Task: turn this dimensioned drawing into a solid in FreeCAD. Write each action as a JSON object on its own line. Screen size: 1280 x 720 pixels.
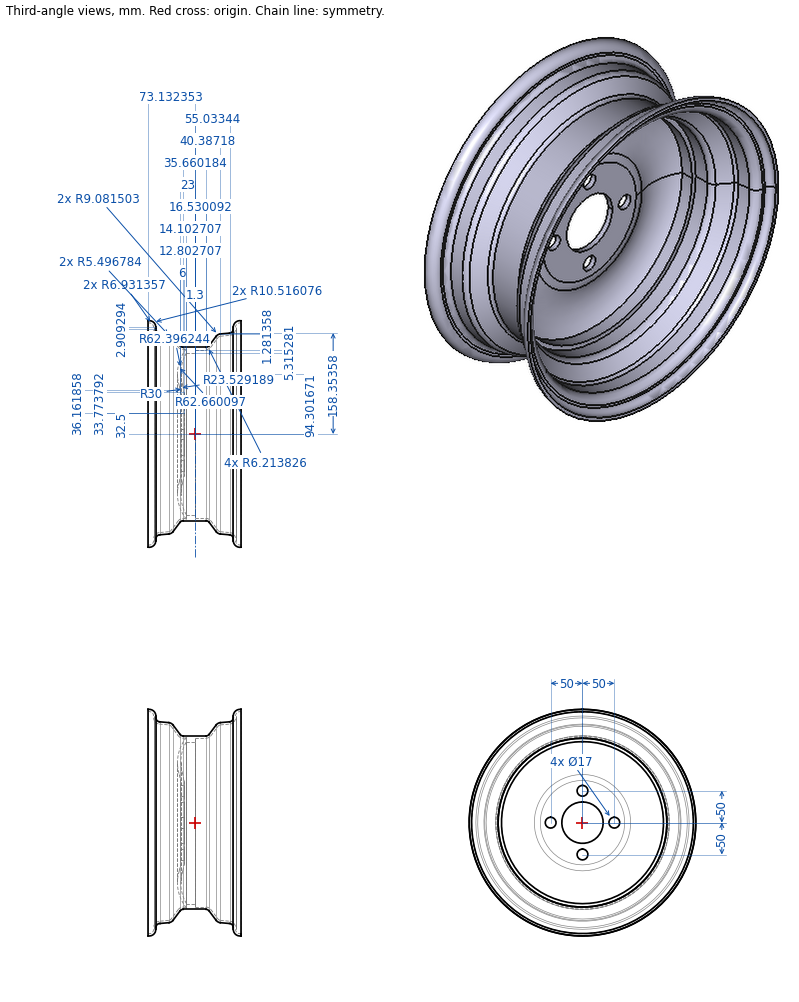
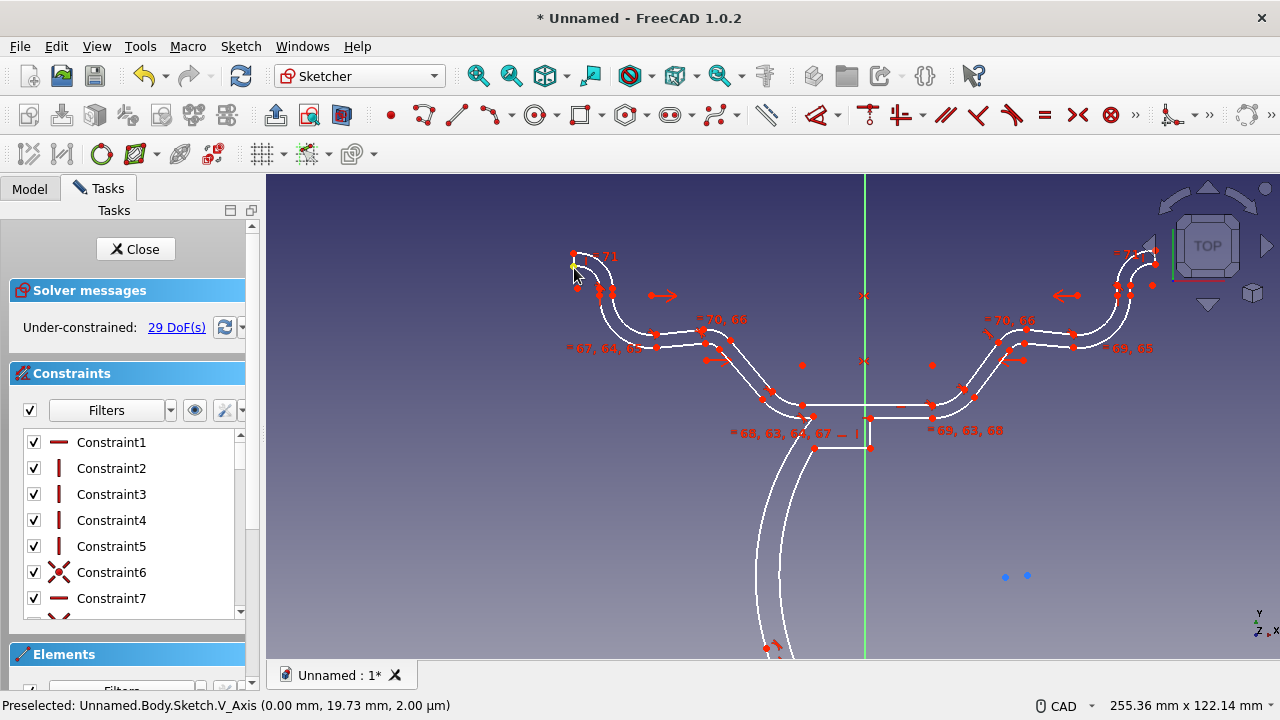
{"action": "left_click", "coordinate": [574, 267]}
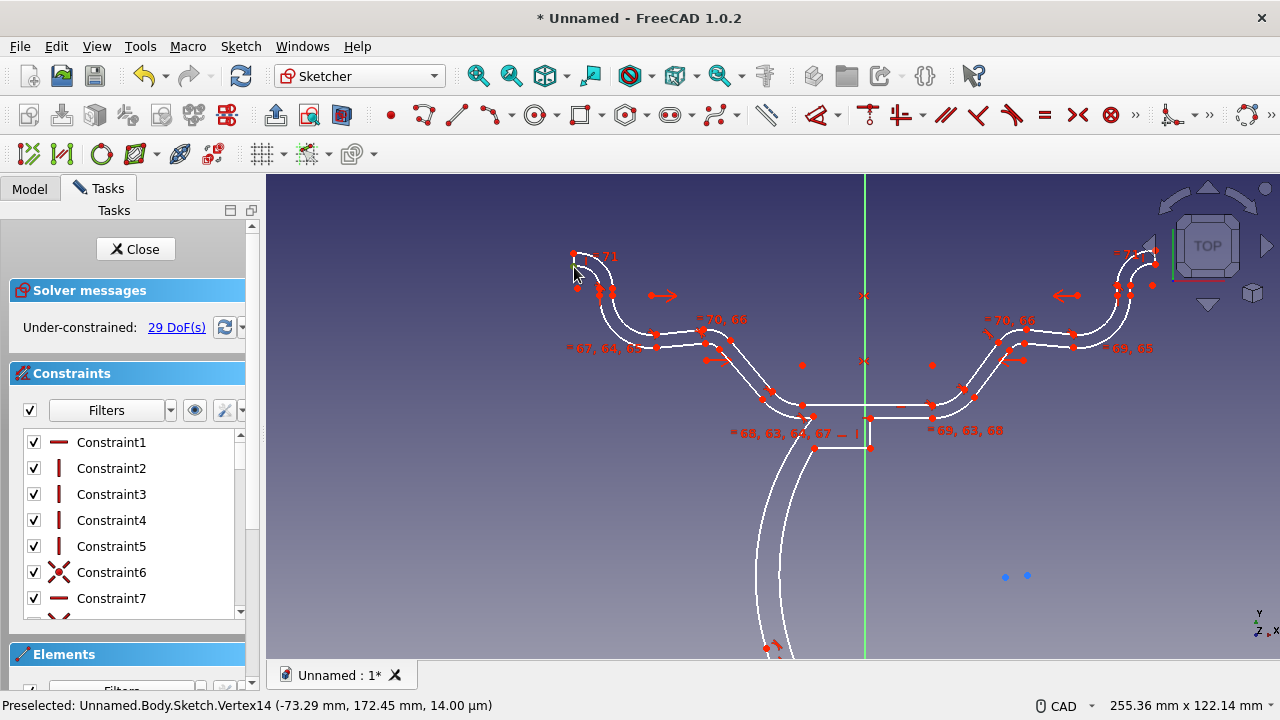
{"action": "scroll", "coordinate": [574, 268], "scroll_direction": "down", "scroll_amount": 4}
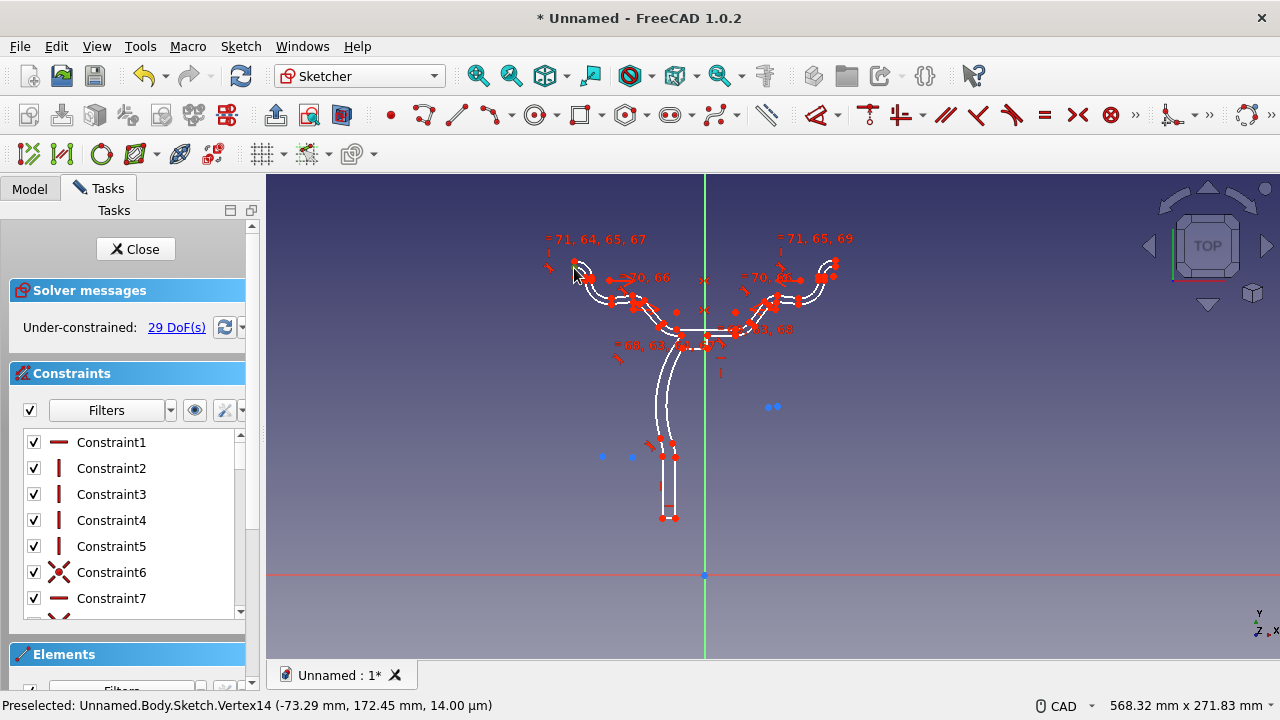
{"action": "scroll", "coordinate": [835, 266], "scroll_direction": "up", "scroll_amount": 4}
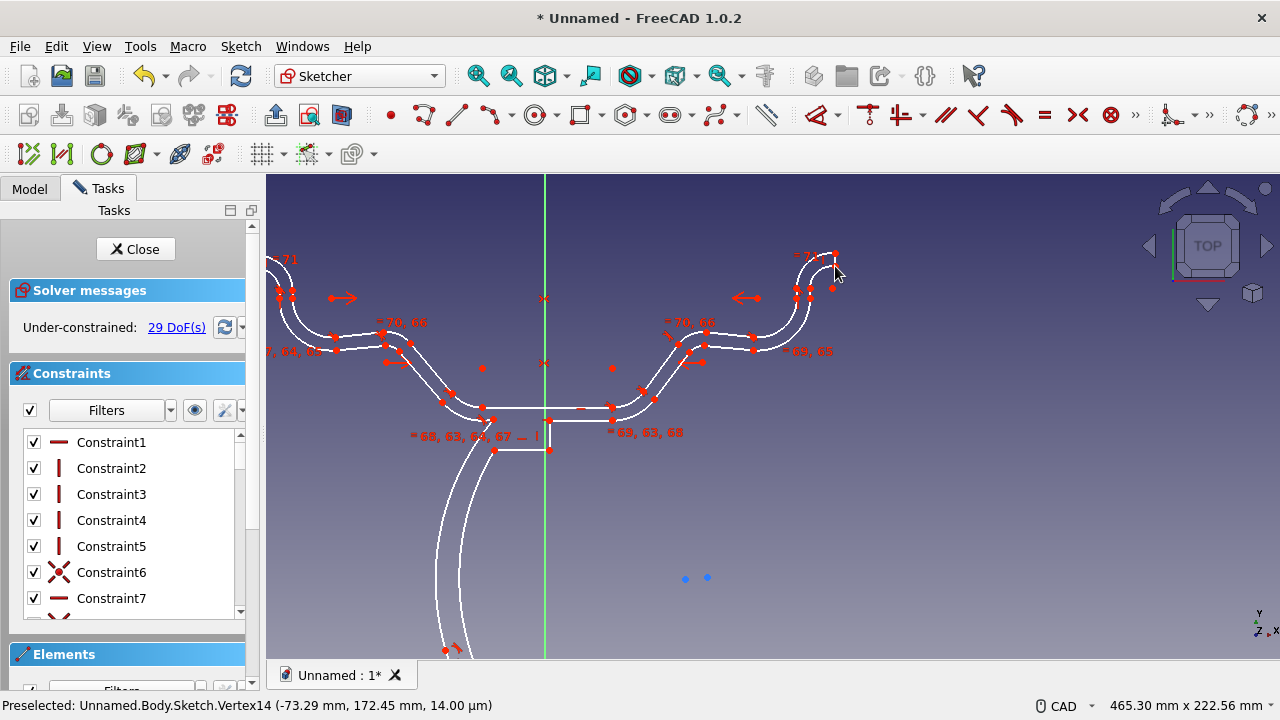
{"action": "left_click", "coordinate": [835, 267]}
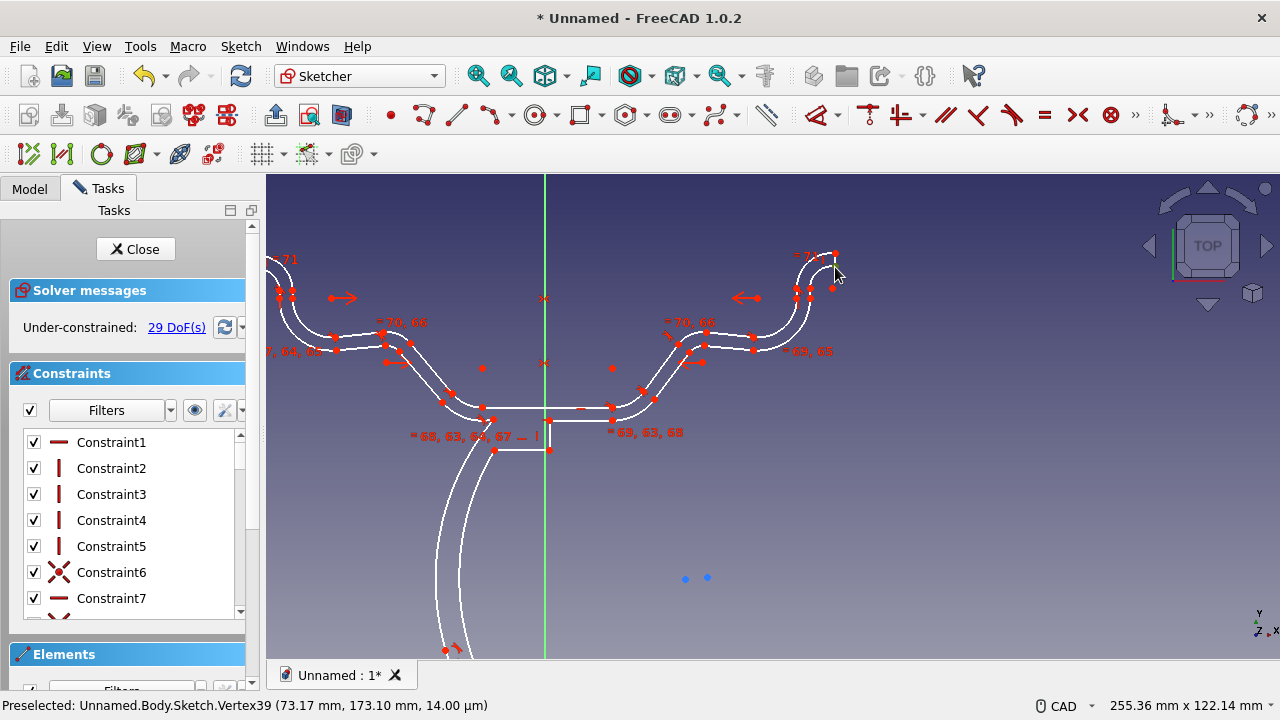
{"action": "left_click", "coordinate": [545, 600]}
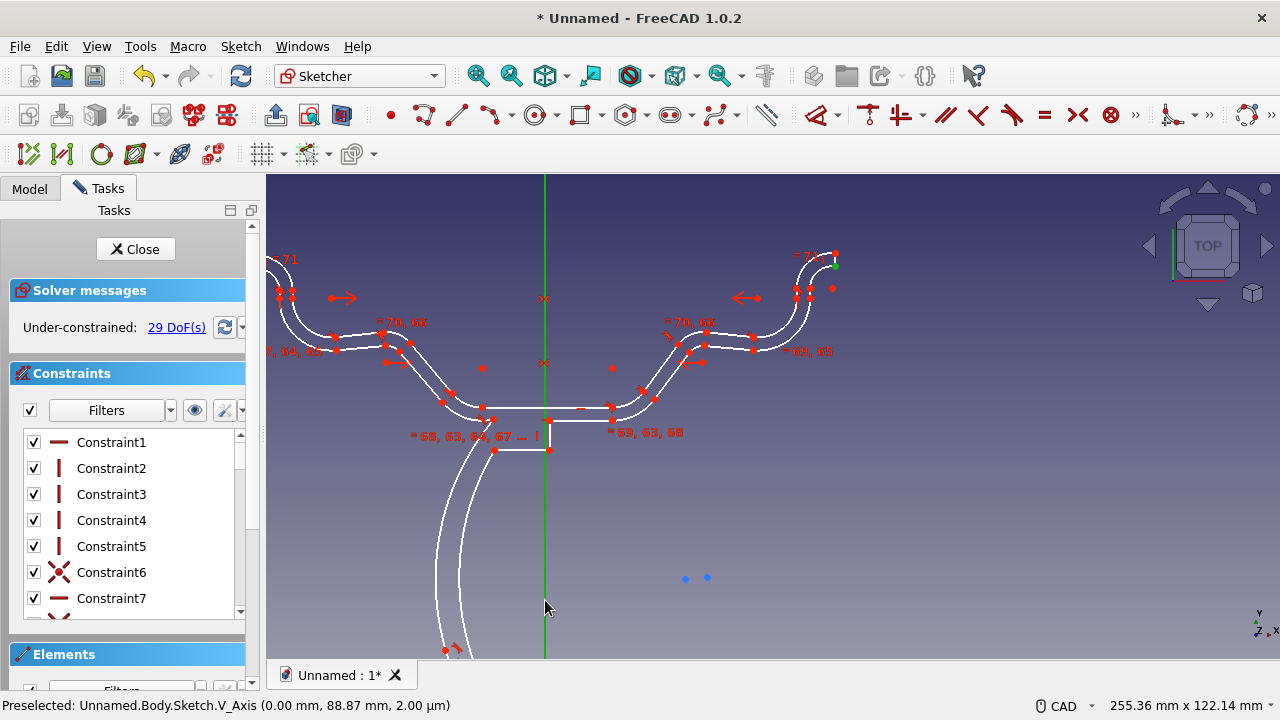
{"action": "key", "text": "s"}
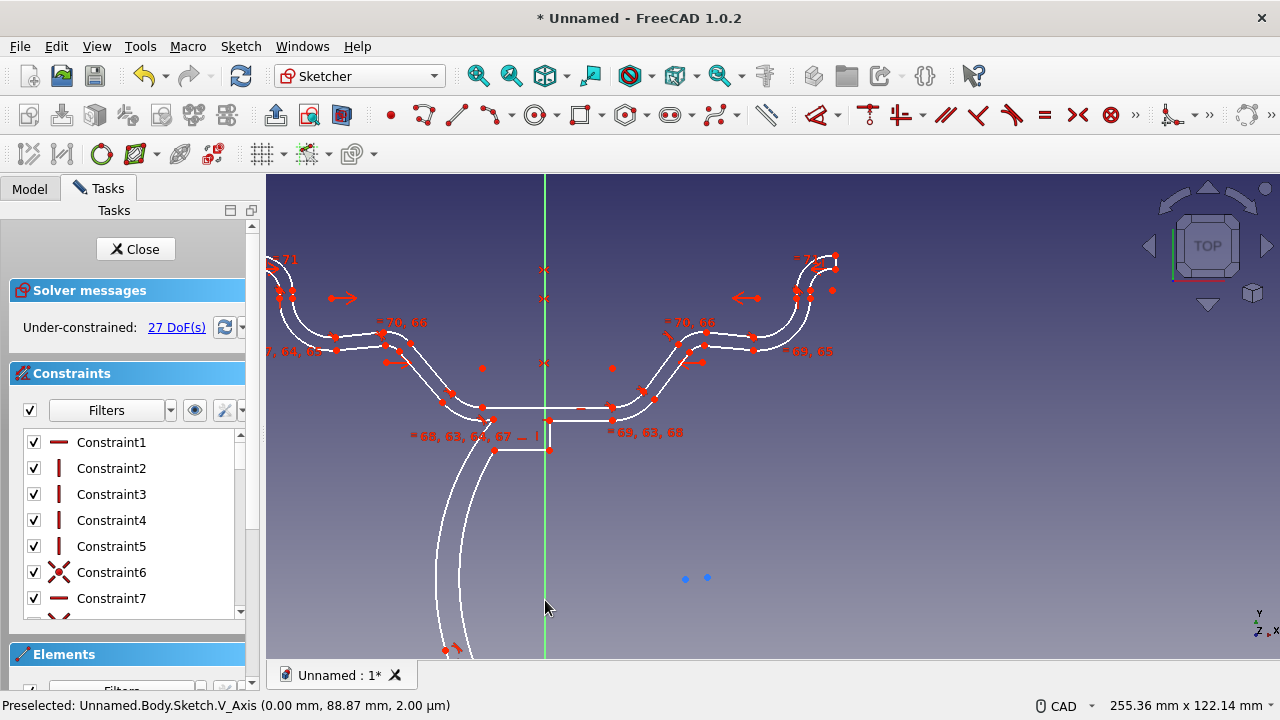
{"action": "left_click", "coordinate": [816, 116]}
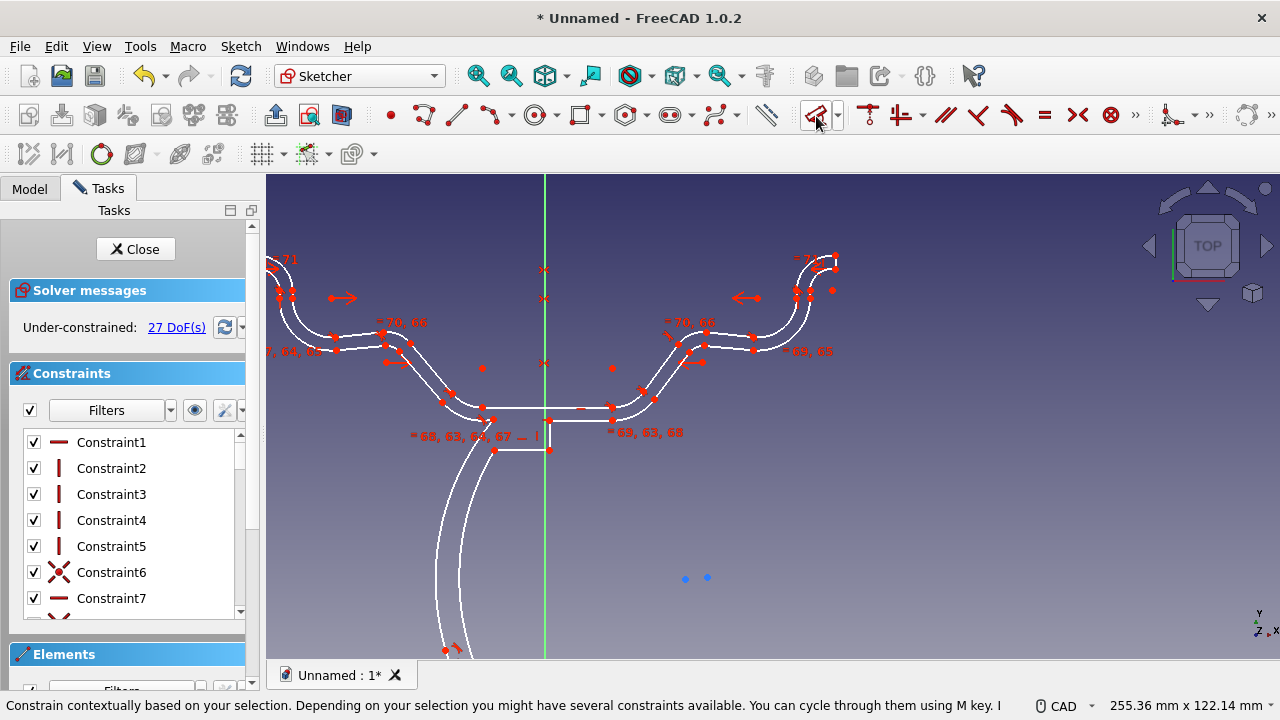
{"action": "scroll", "coordinate": [697, 333], "scroll_direction": "up", "scroll_amount": 2}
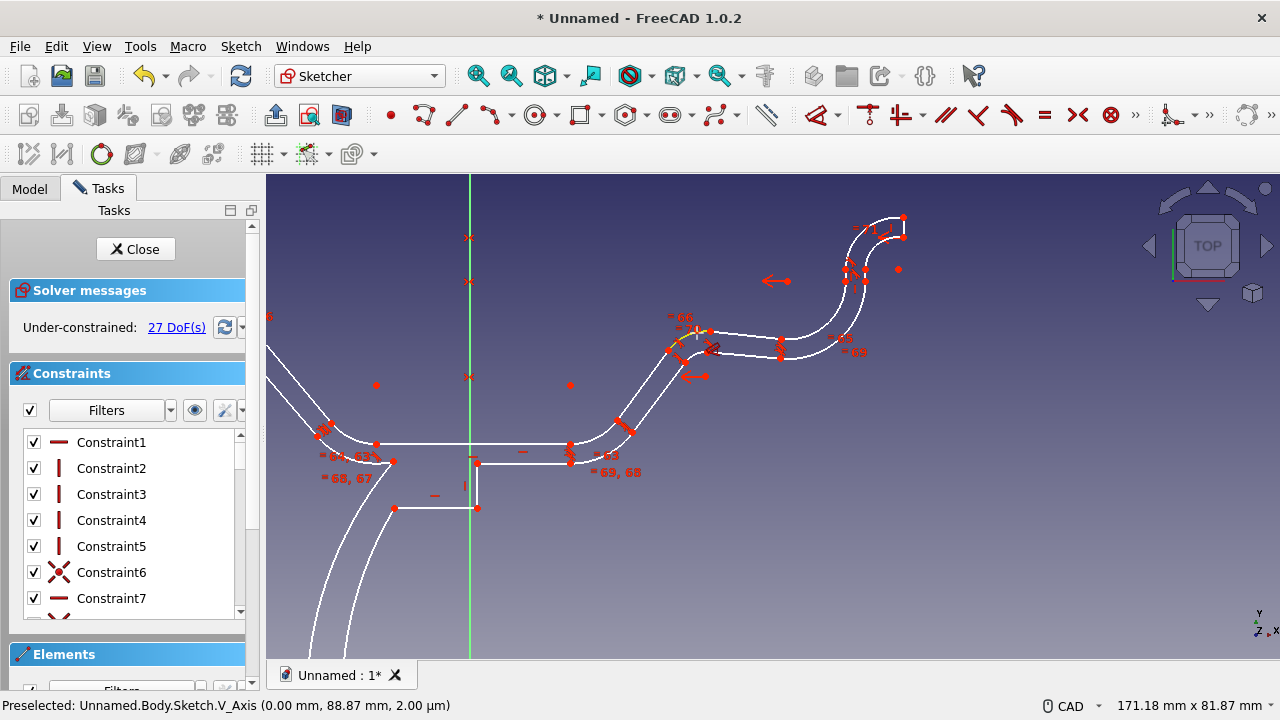
{"action": "left_click", "coordinate": [696, 332]}
{"action": "left_click", "coordinate": [689, 301]}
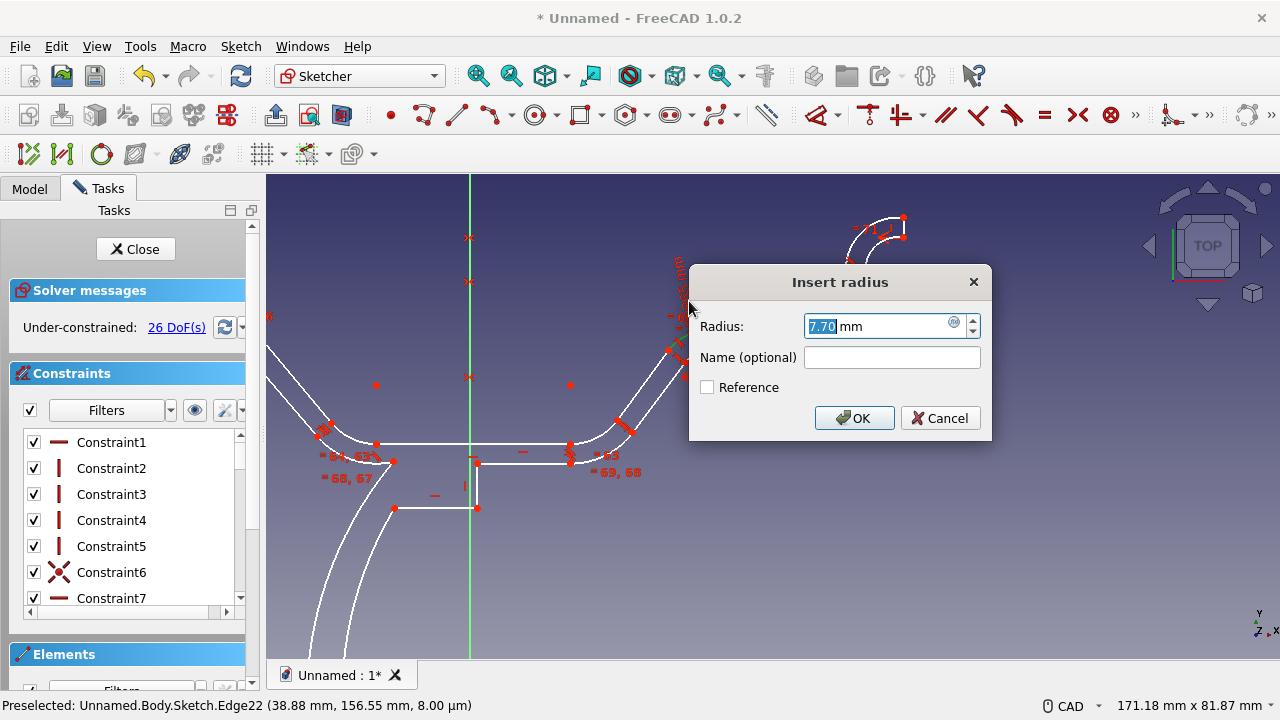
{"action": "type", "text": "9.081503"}
{"action": "key", "text": "Return"}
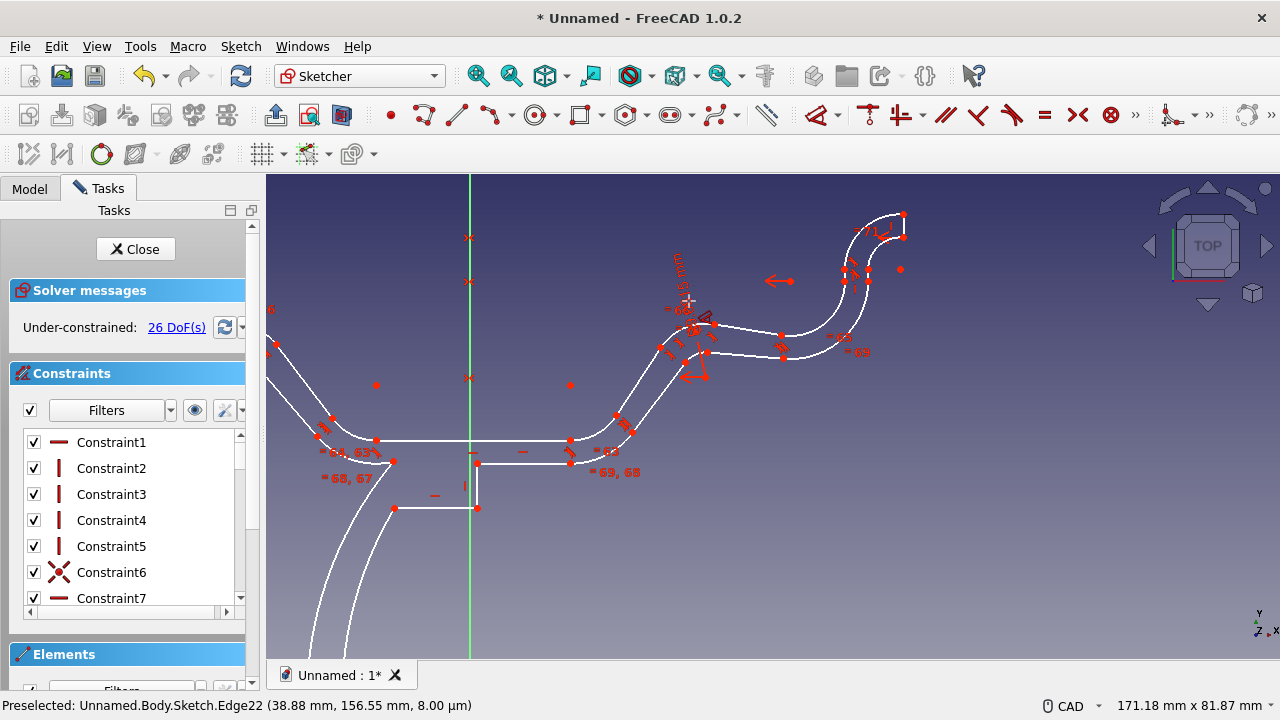
{"action": "left_click", "coordinate": [587, 438]}
{"action": "left_click", "coordinate": [488, 412]}